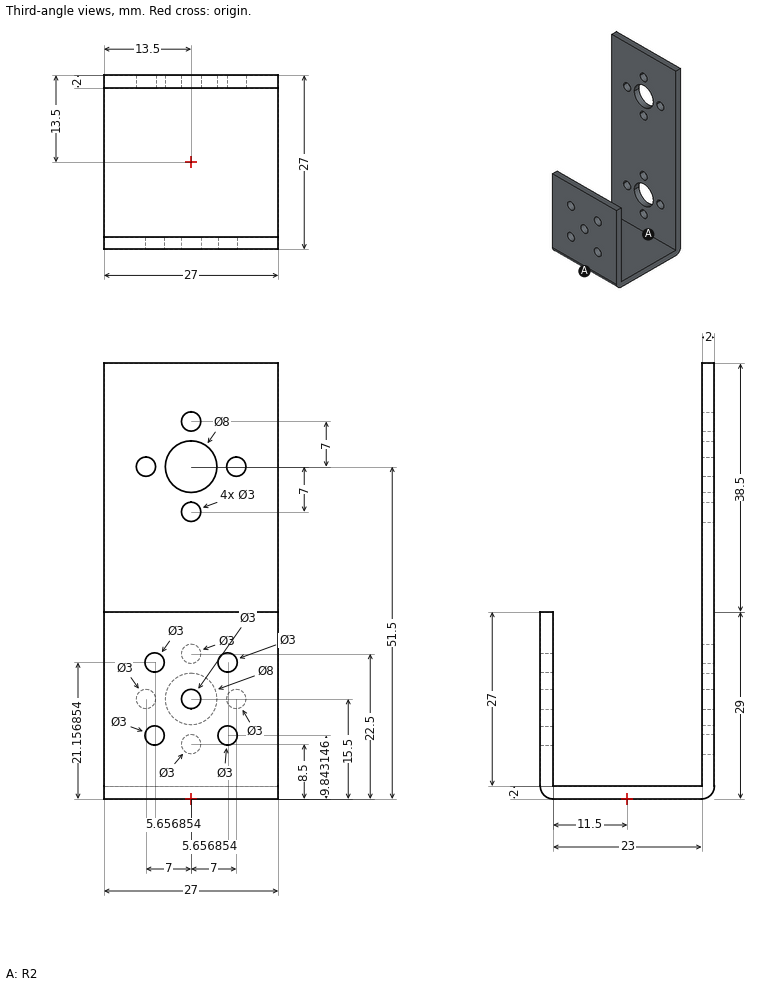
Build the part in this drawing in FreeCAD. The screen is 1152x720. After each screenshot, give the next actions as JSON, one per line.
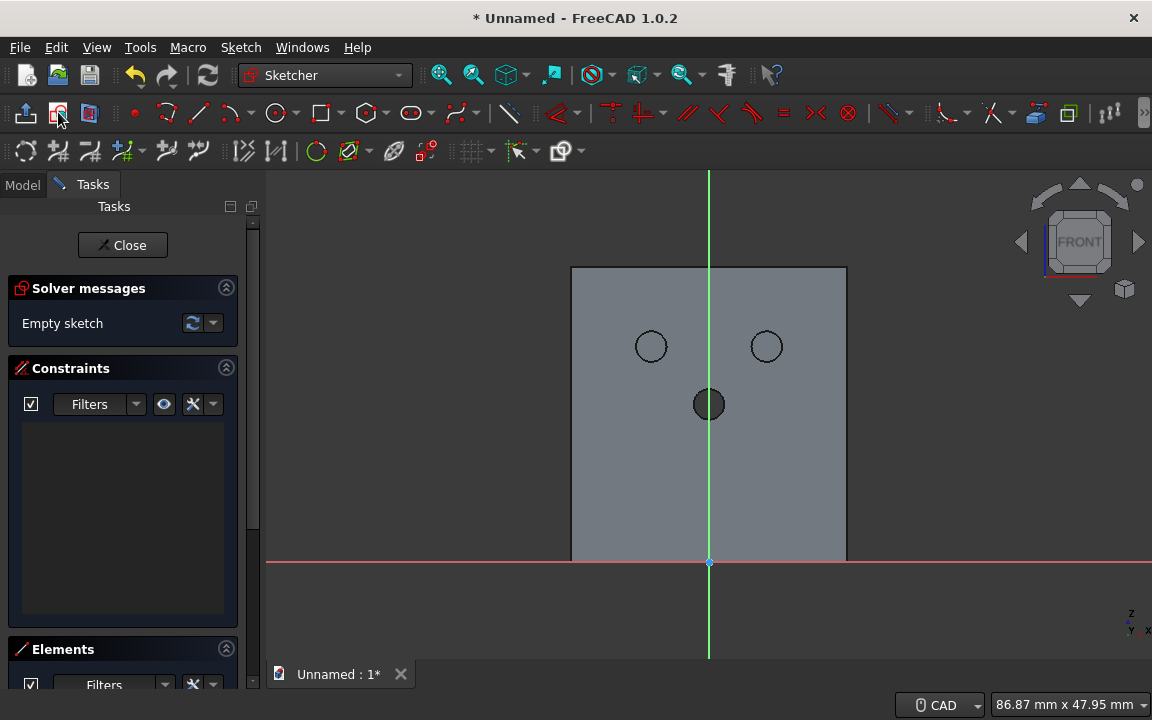
{"action": "scroll", "coordinate": [779, 467], "scroll_direction": "up", "scroll_amount": 12}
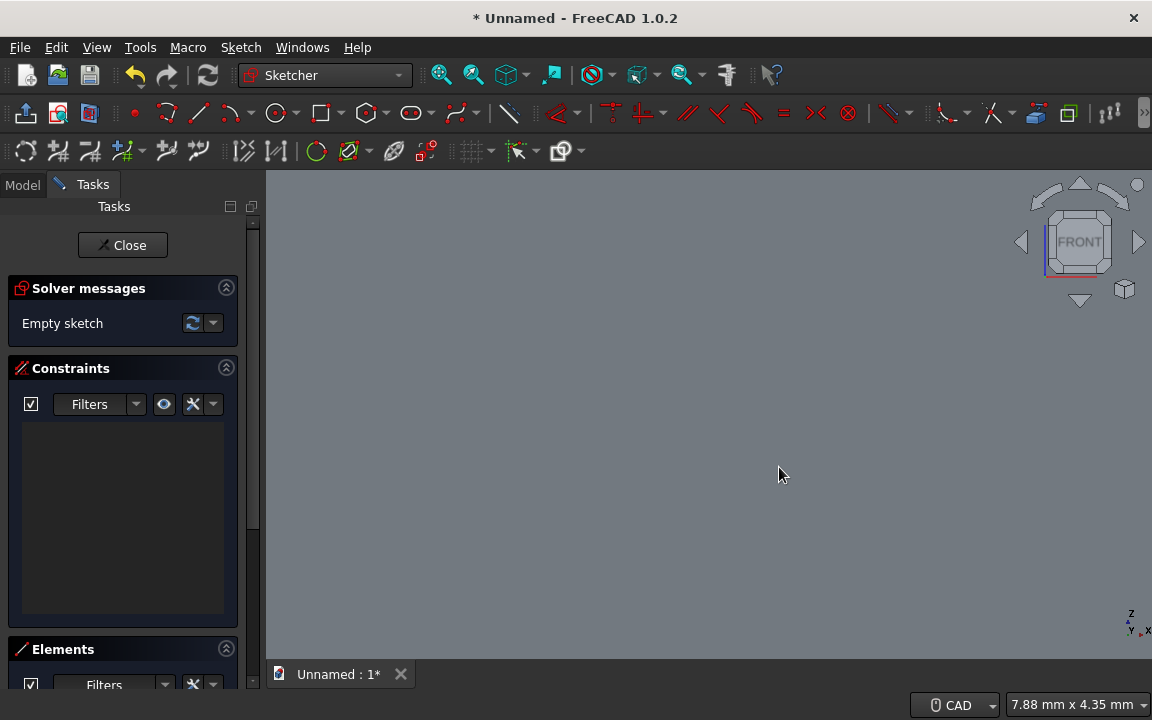
{"action": "key", "text": "g c"}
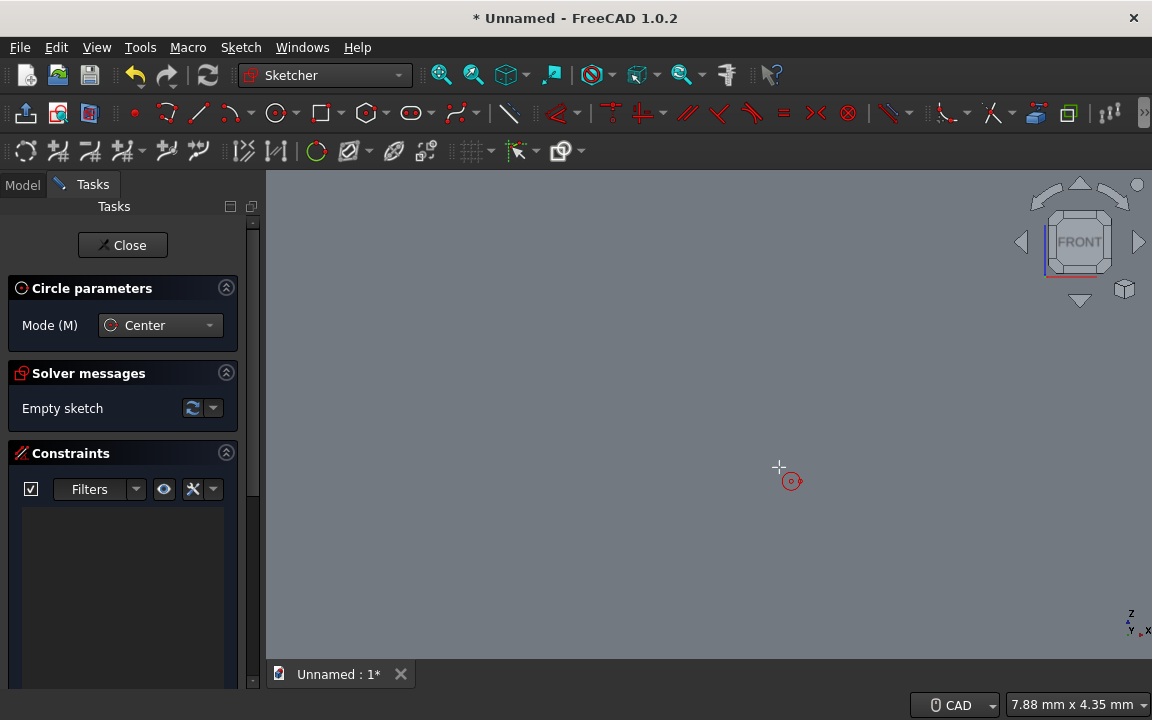
{"action": "left_click", "coordinate": [638, 406]}
{"action": "left_click", "coordinate": [757, 286]}
{"action": "key", "text": "Escape"}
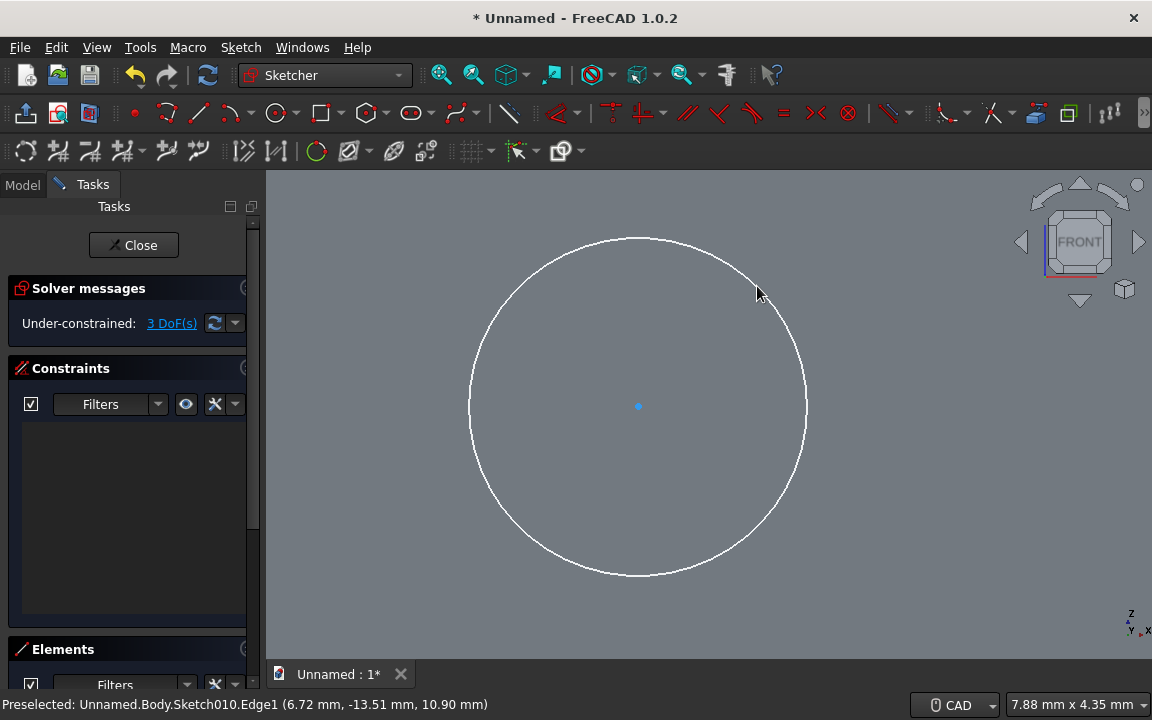
{"action": "key", "text": "d"}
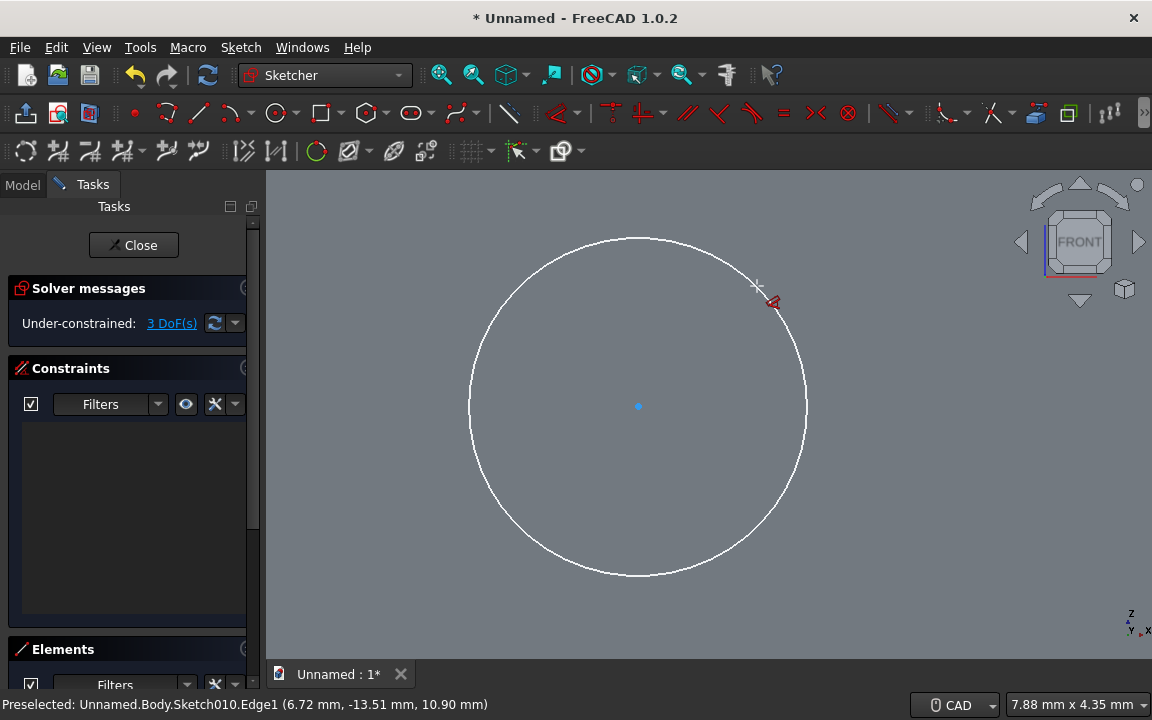
{"action": "left_click", "coordinate": [757, 287]}
{"action": "left_click", "coordinate": [780, 264]}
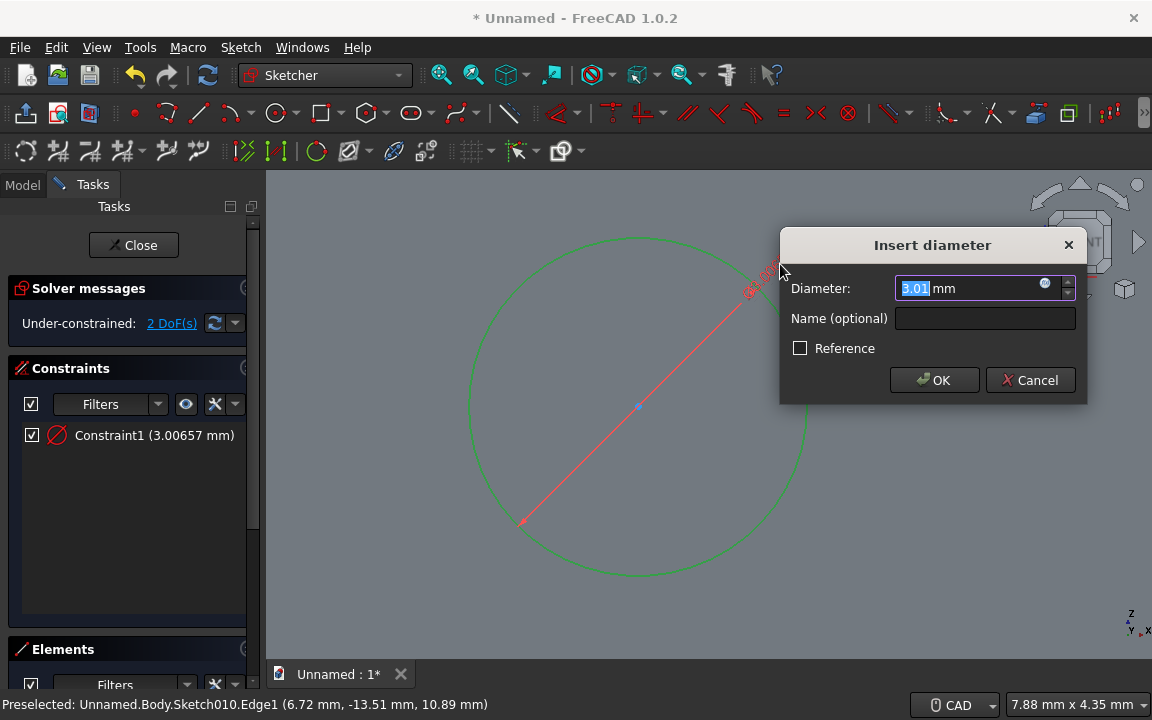
{"action": "type", "text": "3"}
{"action": "key", "text": "Return"}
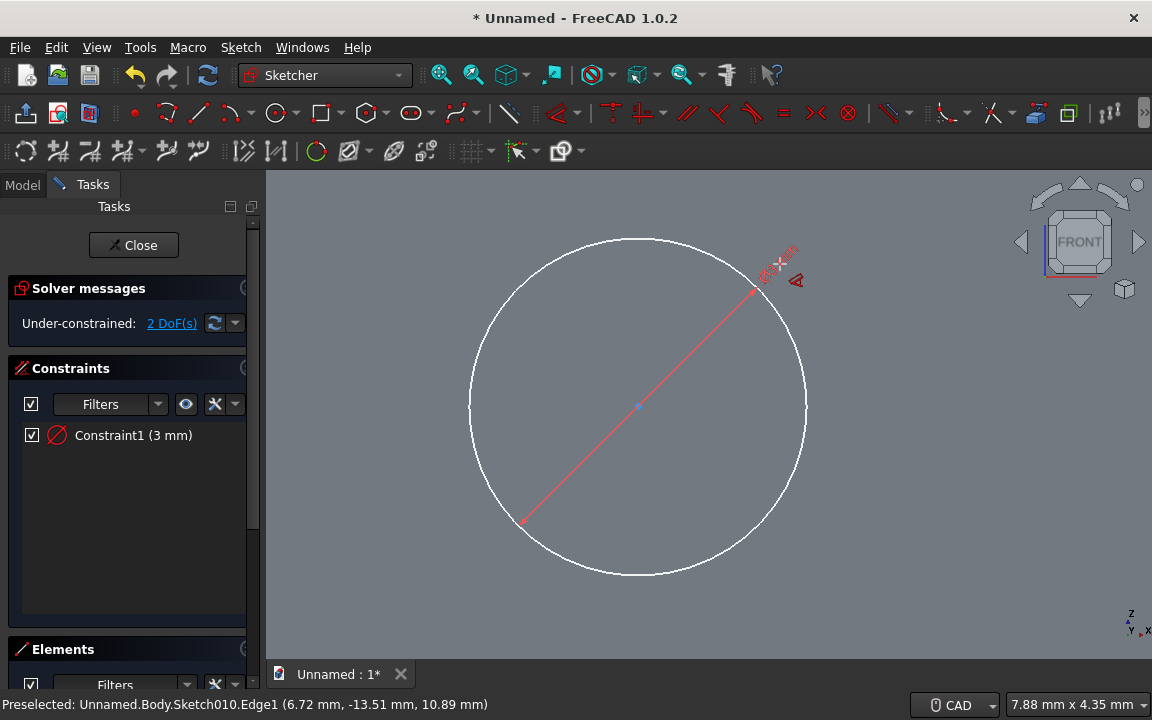
{"action": "left_click", "coordinate": [638, 407]}
{"action": "left_click", "coordinate": [387, 373]}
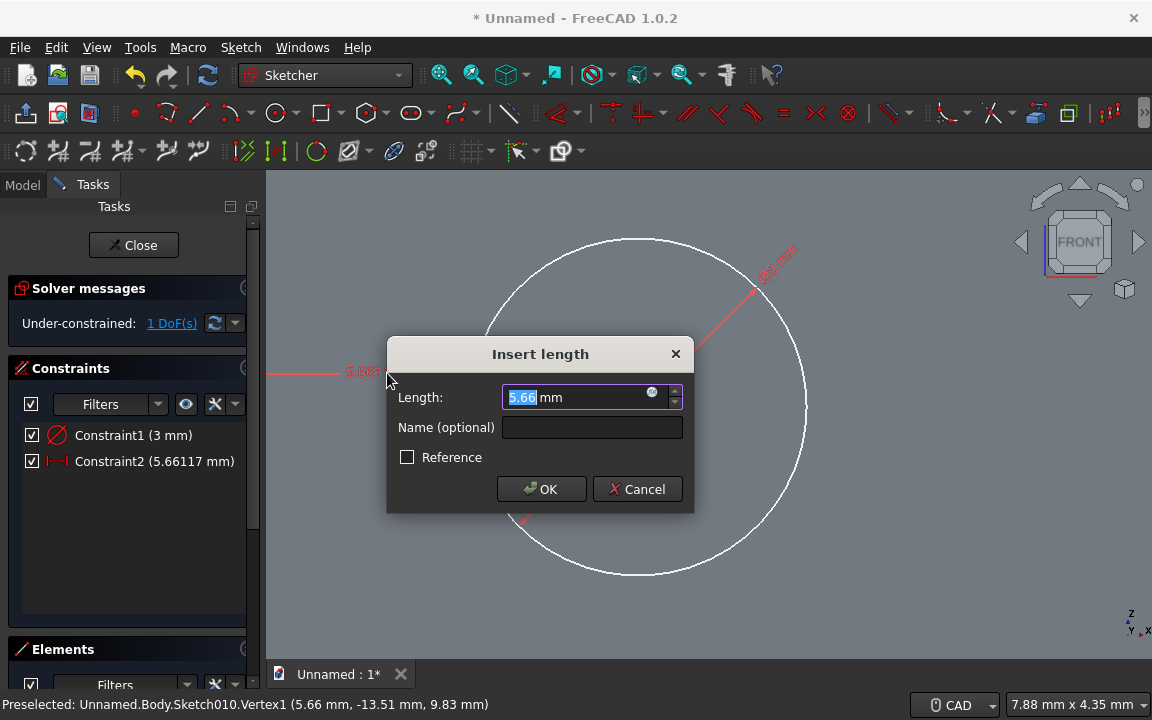
{"action": "type", "text": "5.656854"}
{"action": "key", "text": "Return"}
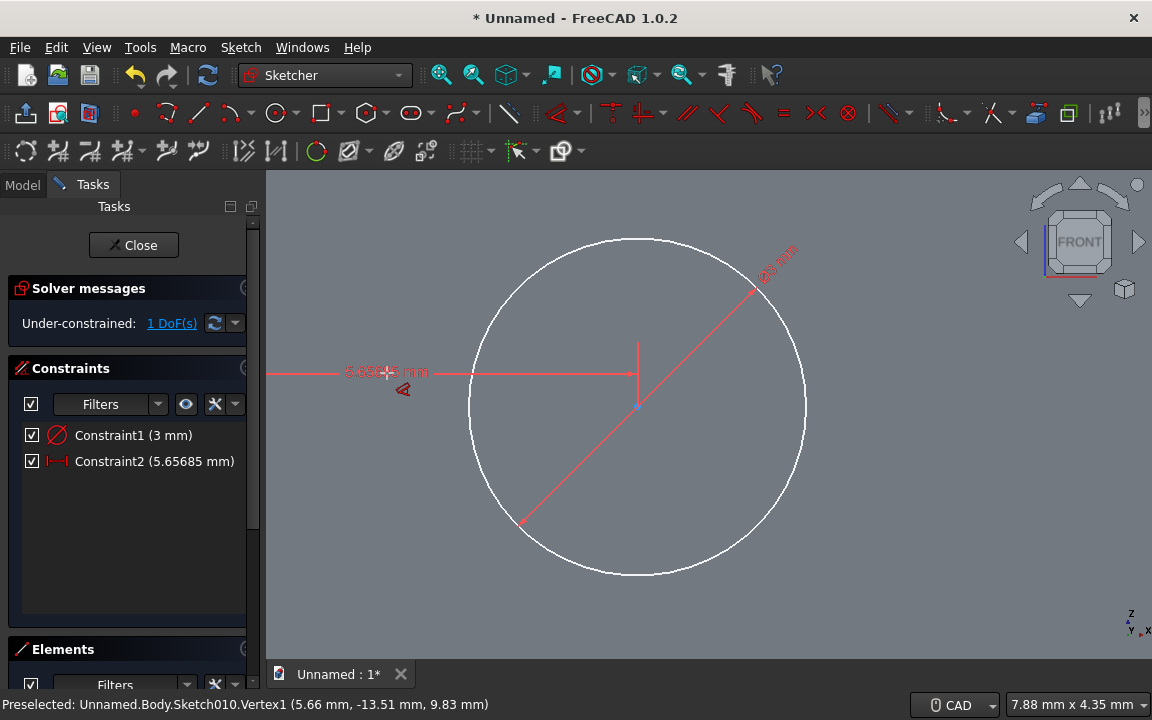
{"action": "left_click", "coordinate": [638, 407]}
{"action": "left_click", "coordinate": [672, 519]}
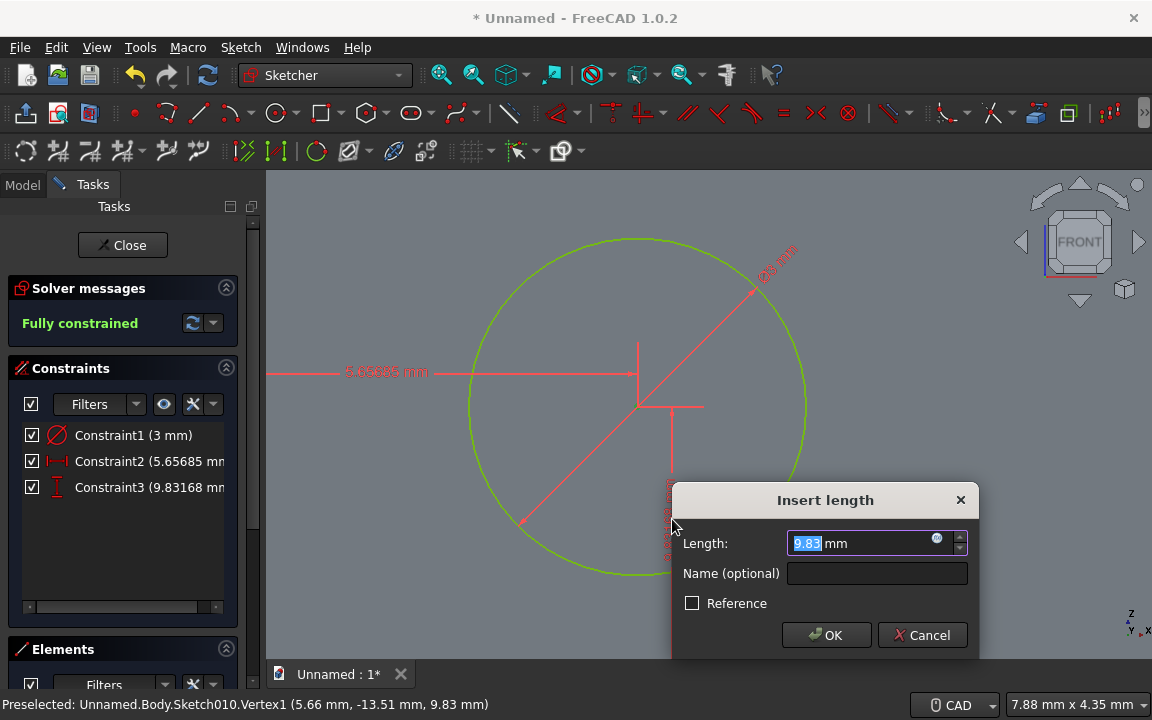
{"action": "type", "text": "9.843146"}
{"action": "key", "text": "Return"}
{"action": "key", "text": "Escape"}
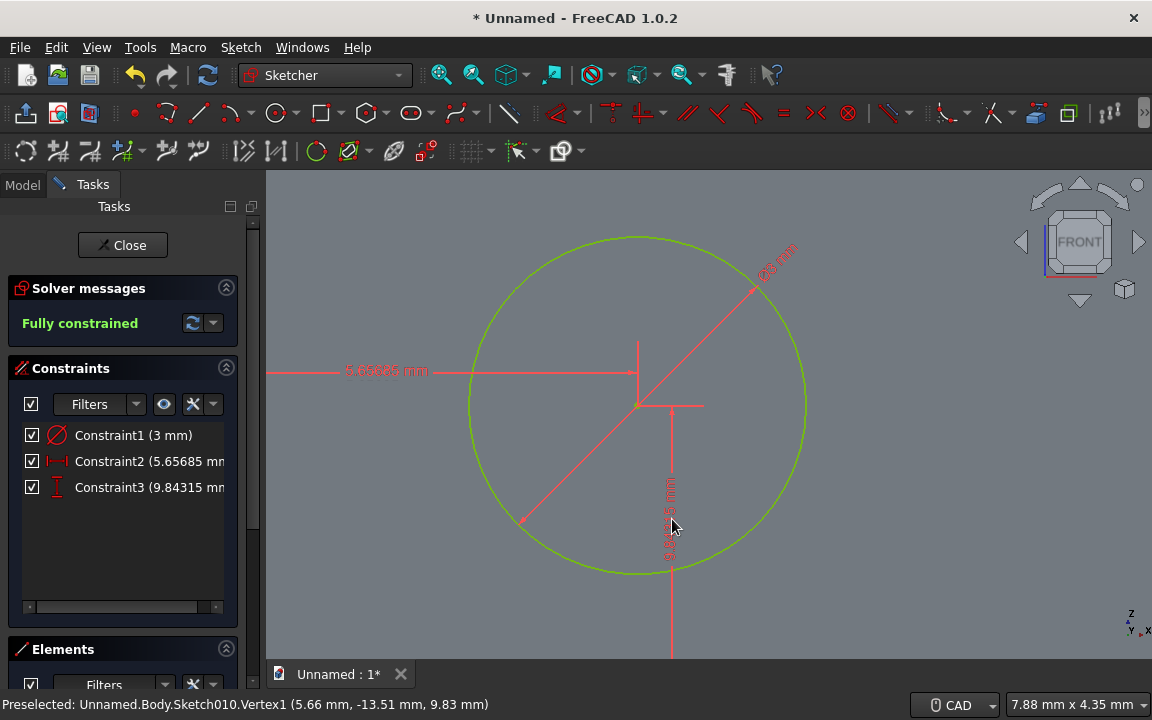
{"action": "left_click", "coordinate": [123, 245]}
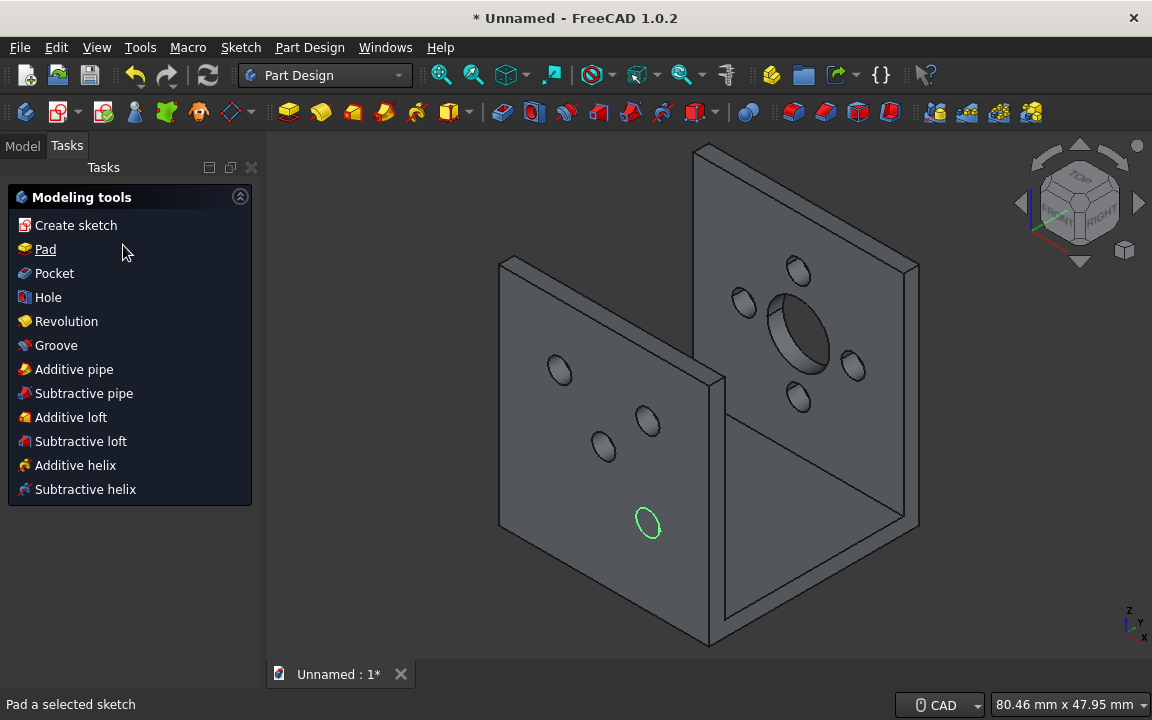
{"action": "left_click", "coordinate": [504, 112]}